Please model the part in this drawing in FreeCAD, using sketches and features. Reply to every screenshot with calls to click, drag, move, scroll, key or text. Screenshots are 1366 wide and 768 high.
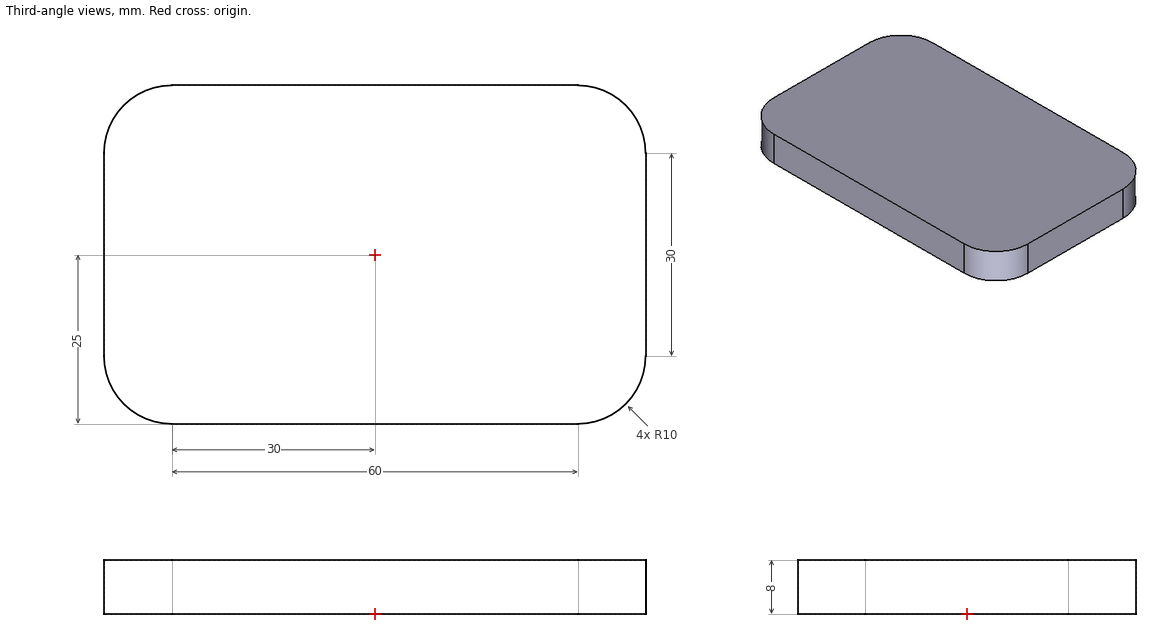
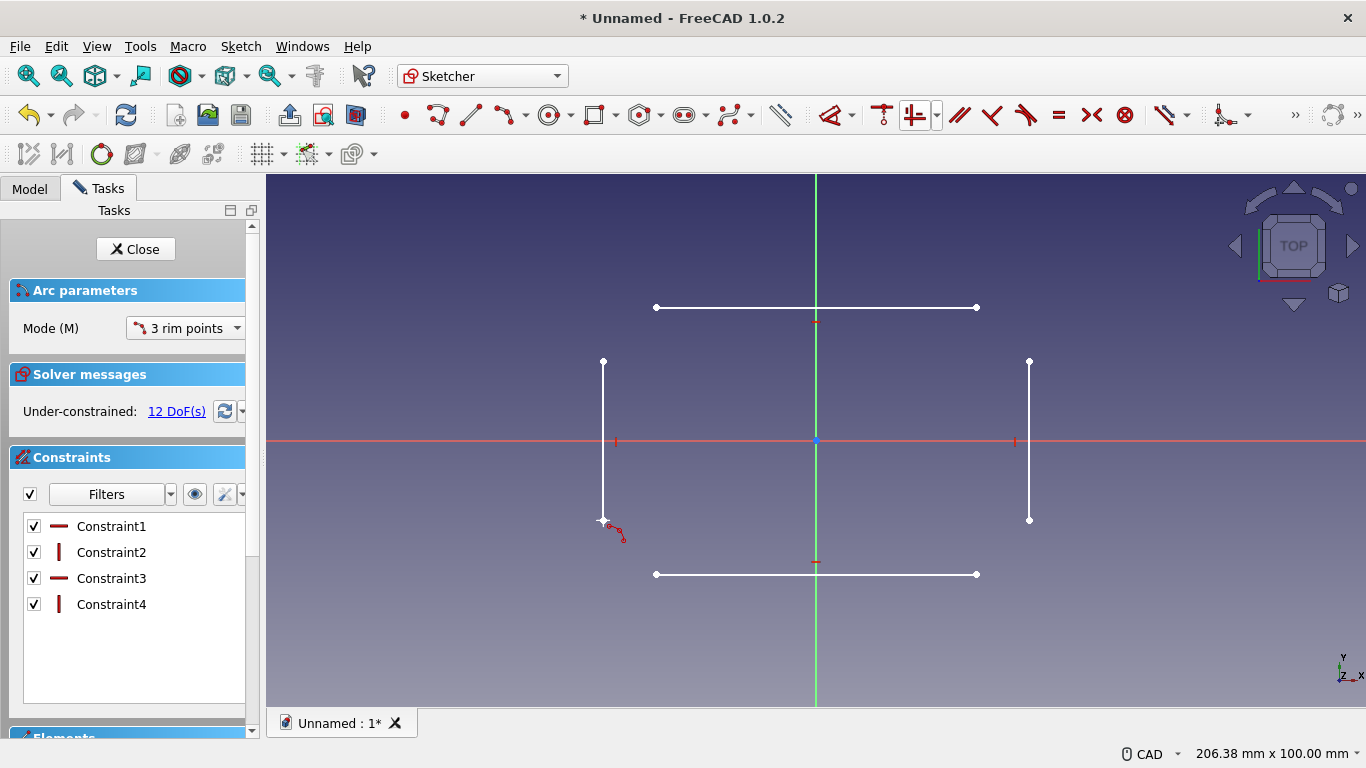
click(976, 575)
click(1029, 521)
click(1014, 558)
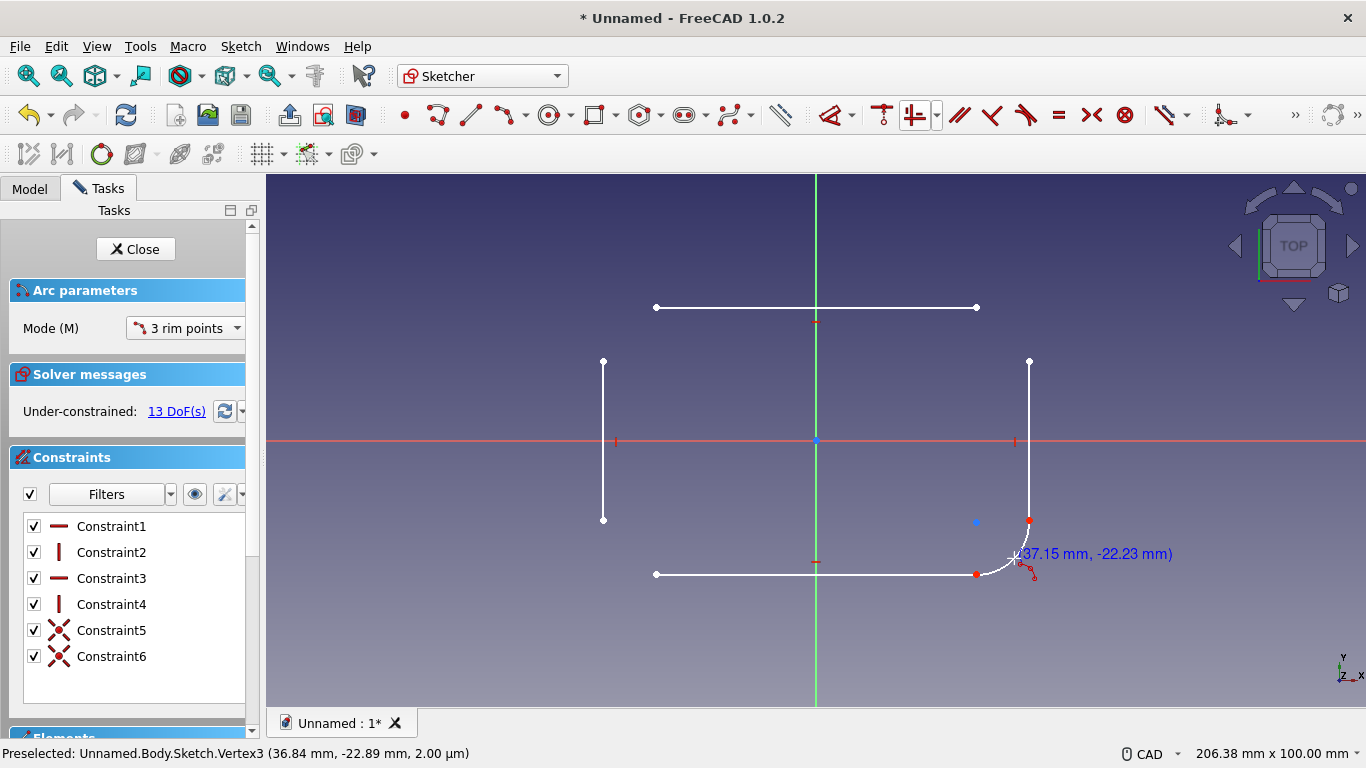
click(1029, 362)
click(976, 308)
click(1014, 323)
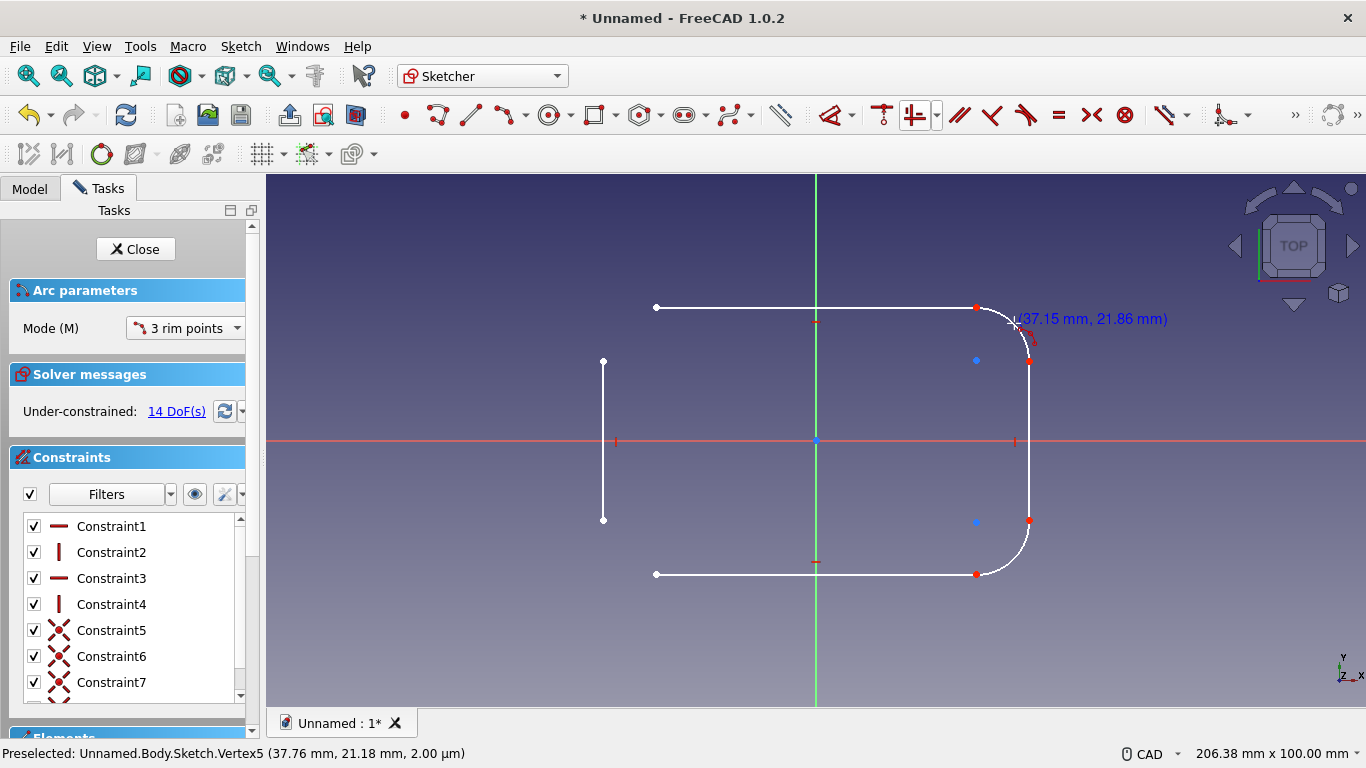
click(656, 308)
click(603, 362)
click(618, 323)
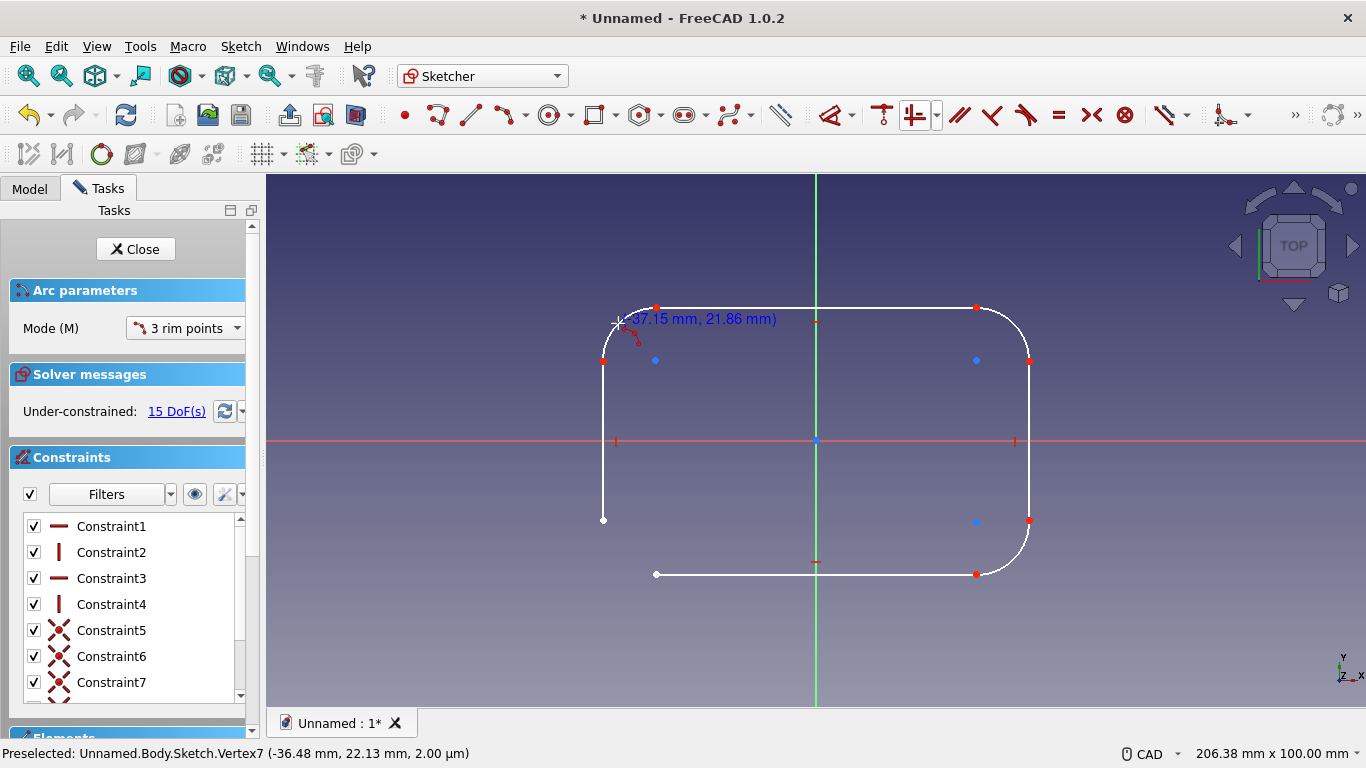
click(603, 521)
click(656, 575)
click(618, 558)
key(Escape)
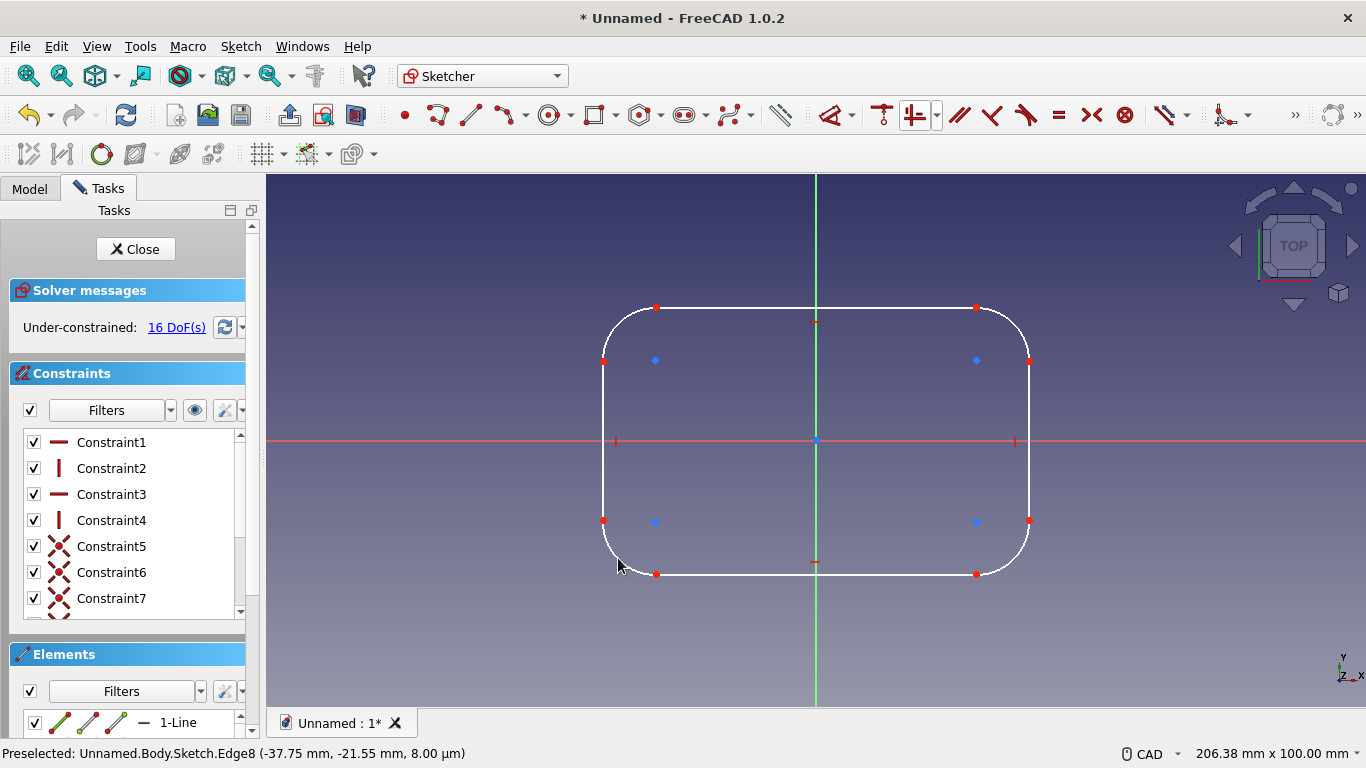
click(752, 575)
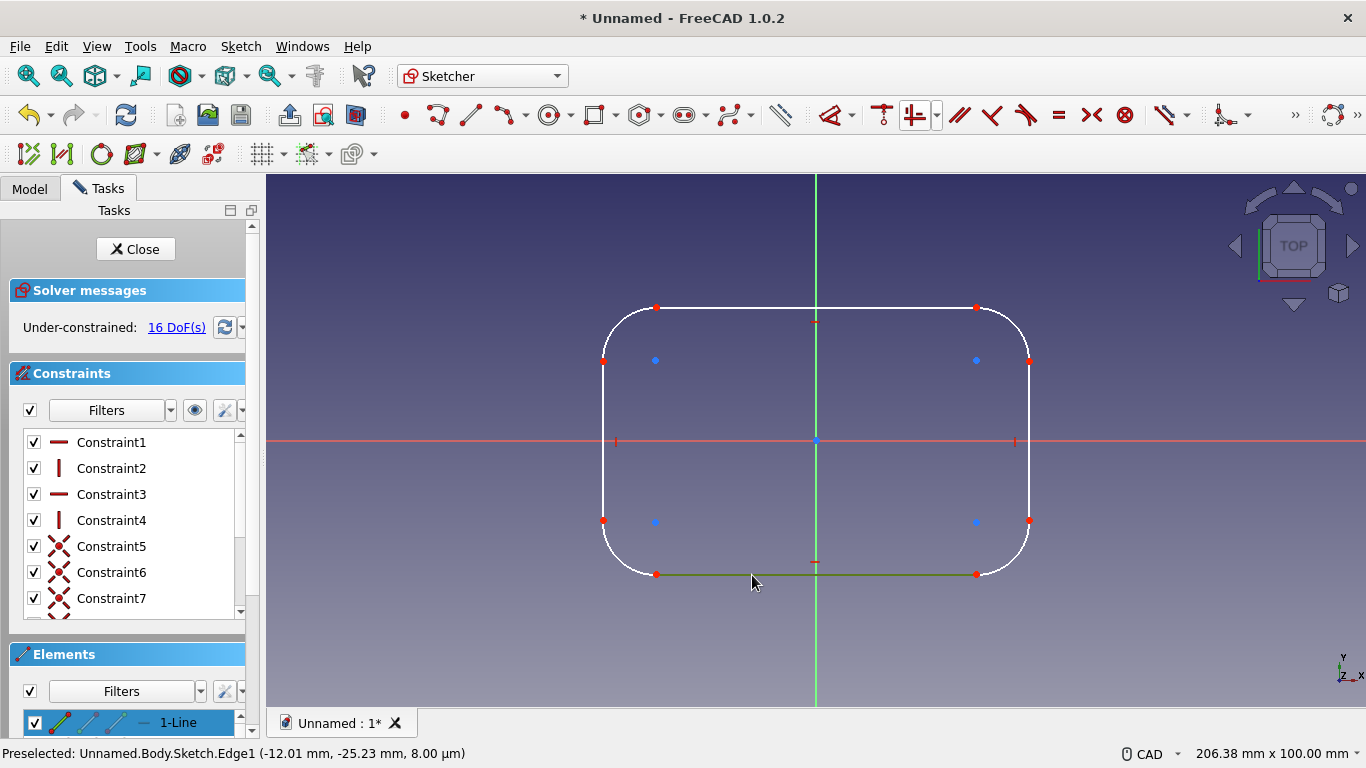
click(1000, 569)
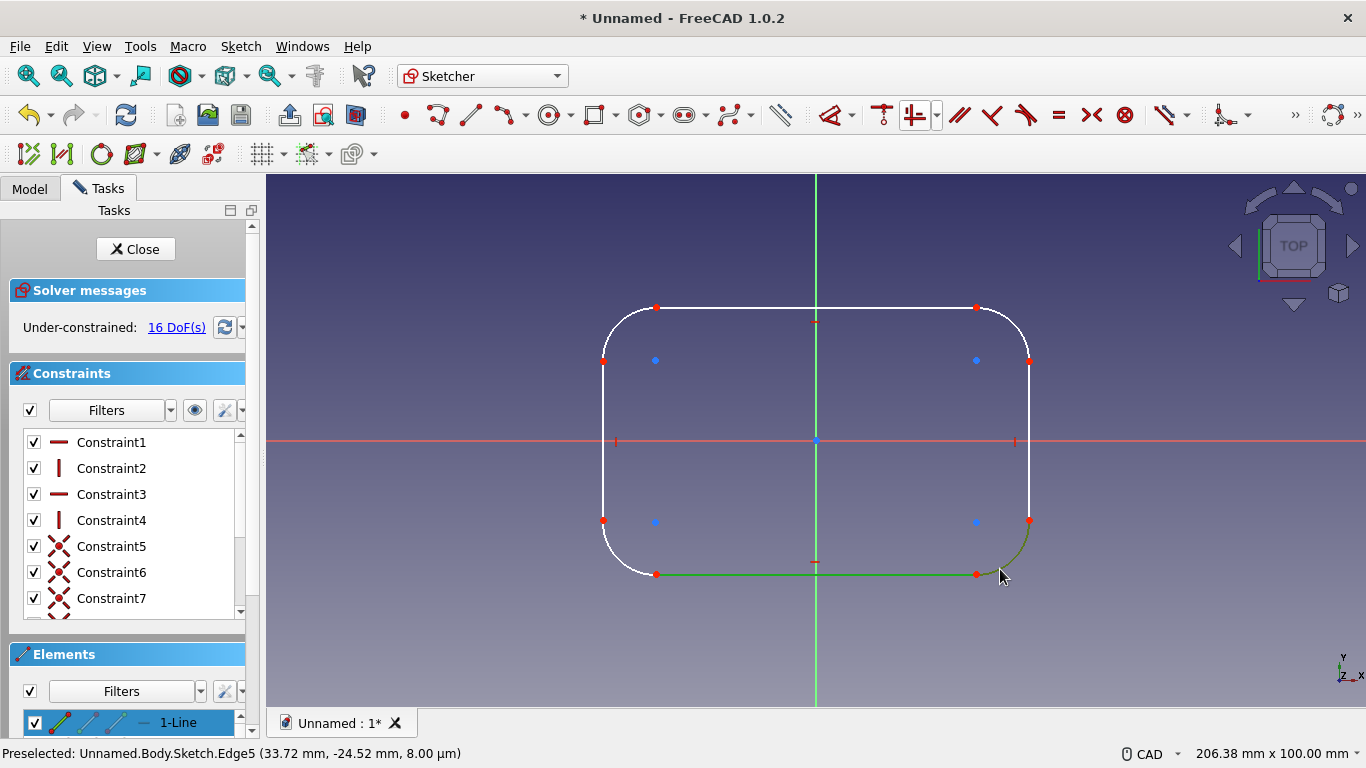
key(t)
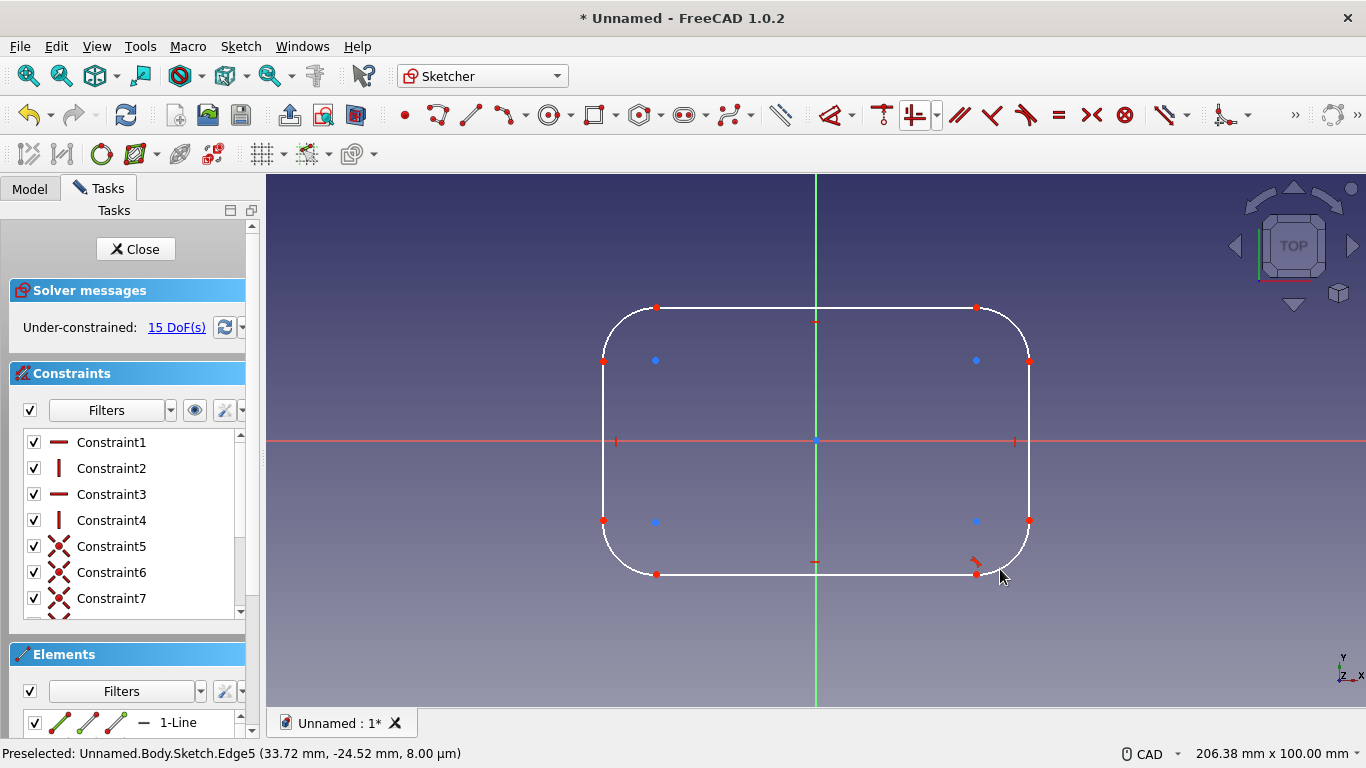
click(752, 575)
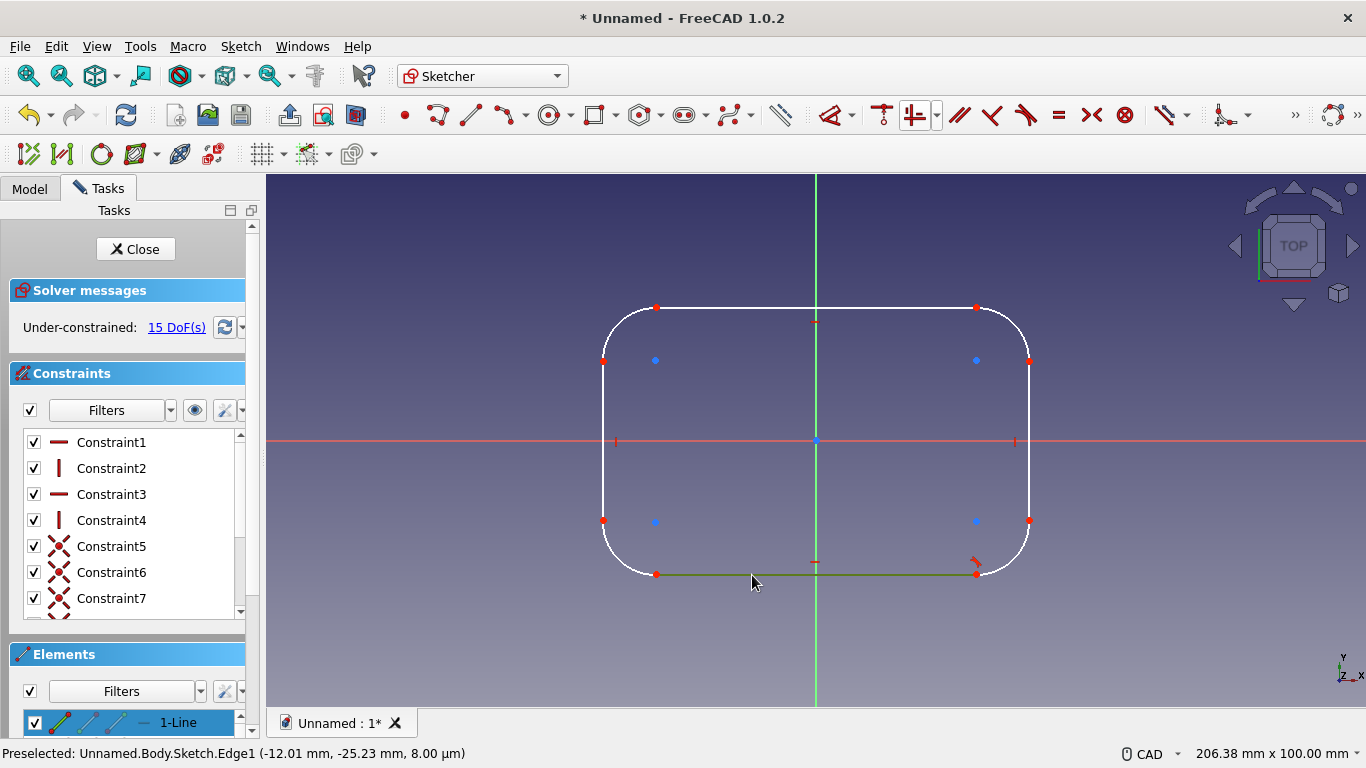
click(608, 545)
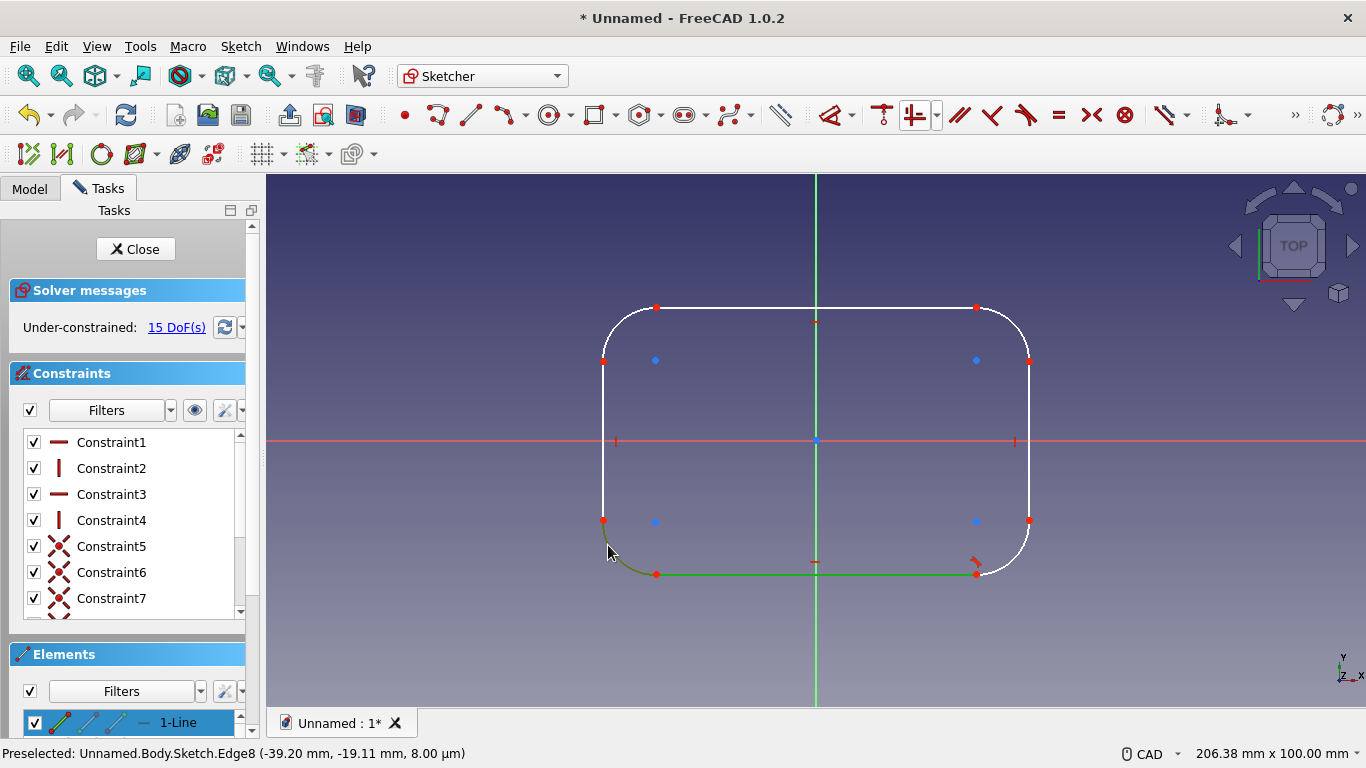
click(1026, 116)